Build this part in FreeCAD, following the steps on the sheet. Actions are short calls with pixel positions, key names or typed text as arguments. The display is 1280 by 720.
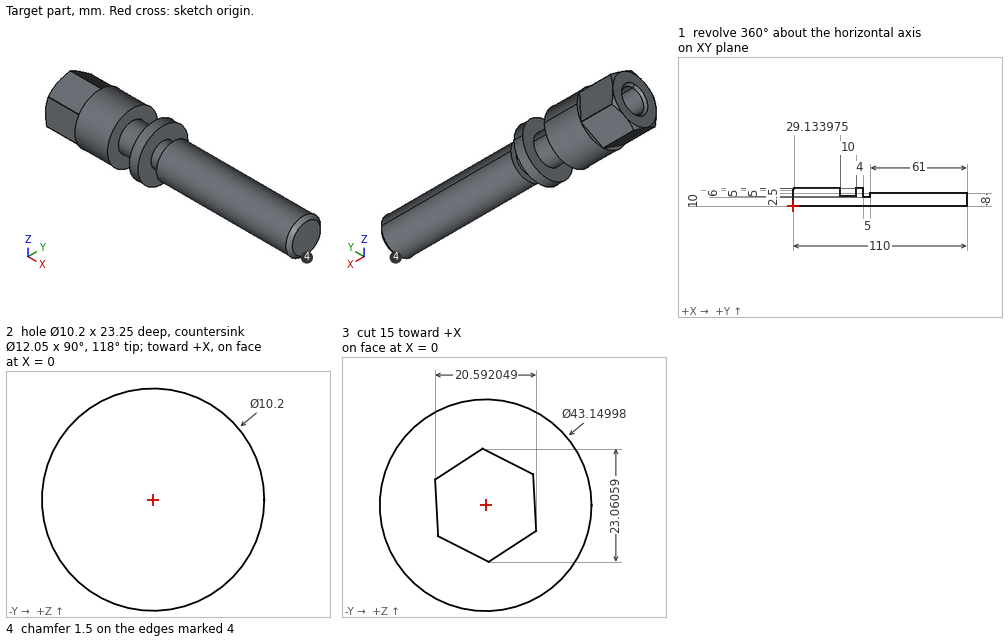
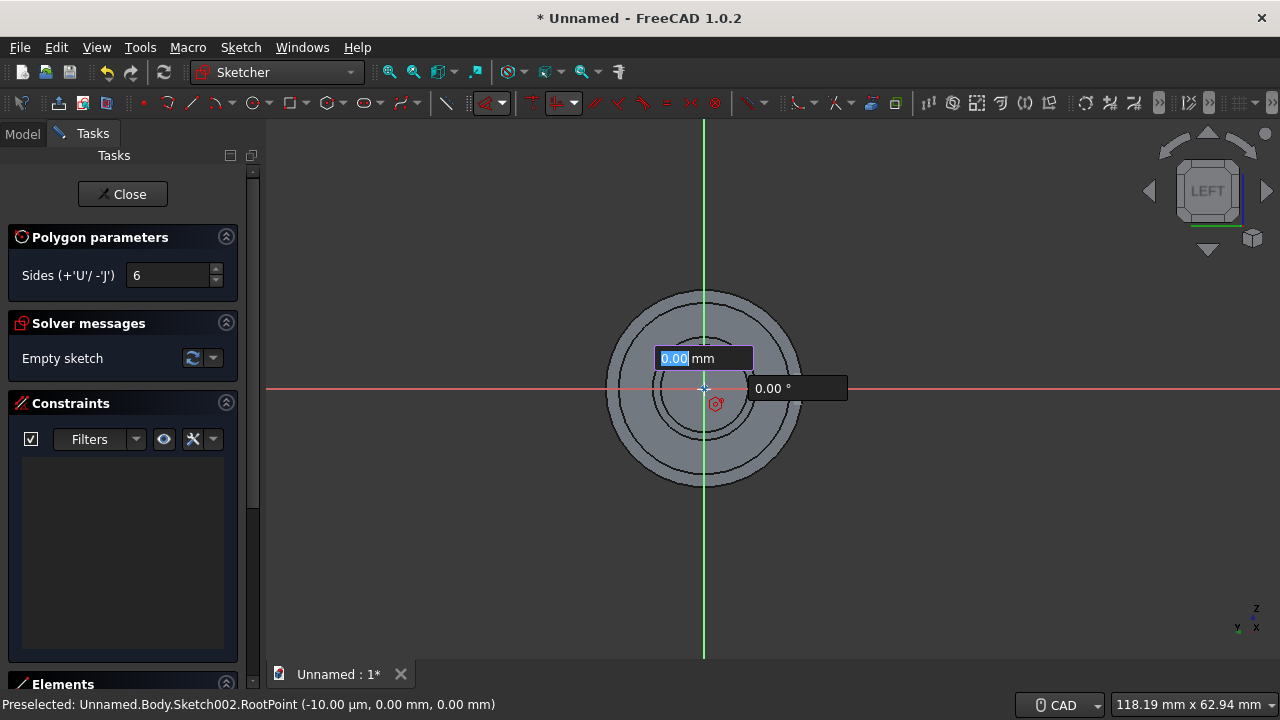
click(621, 443)
right_click(621, 443)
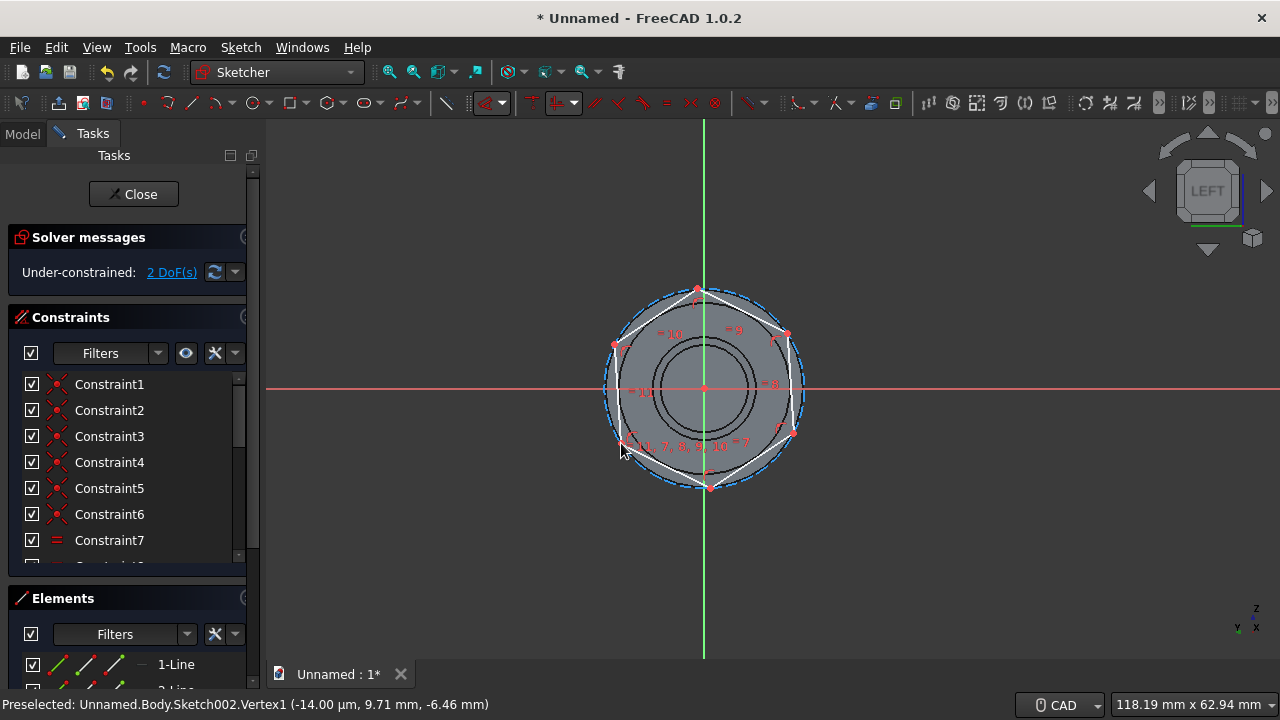
key(g)
key(c)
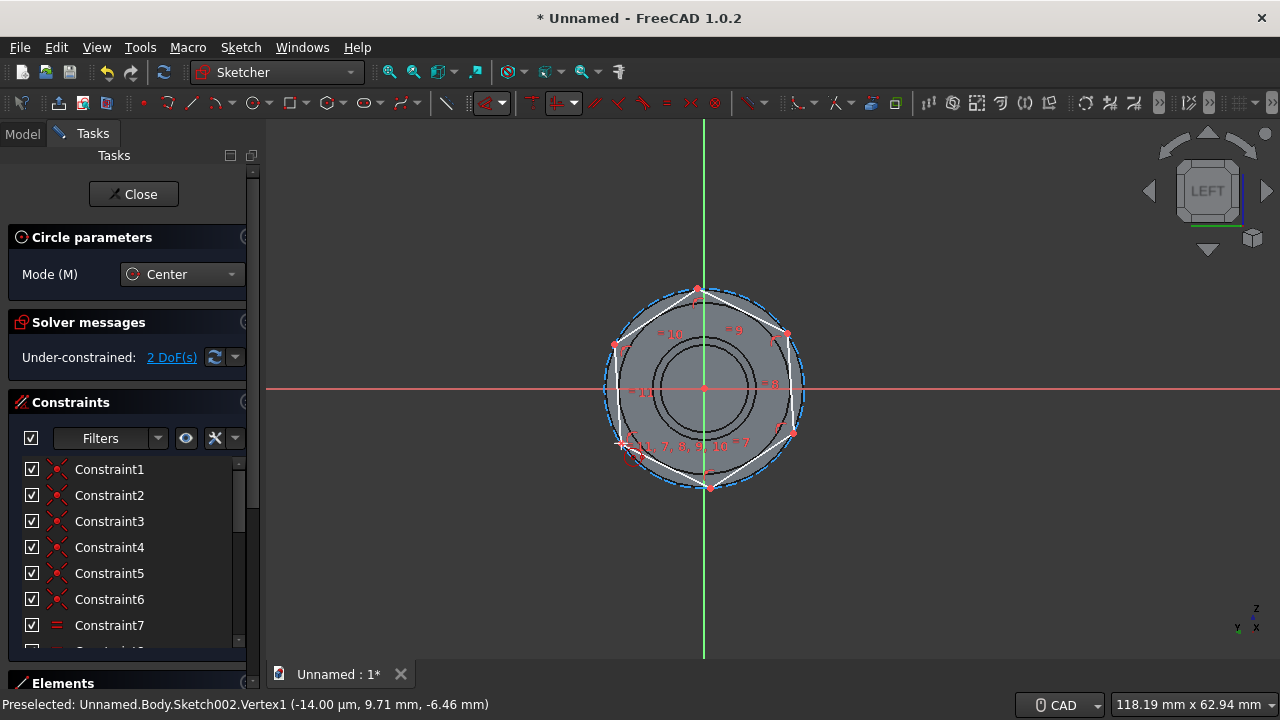
click(704, 389)
move(835, 258)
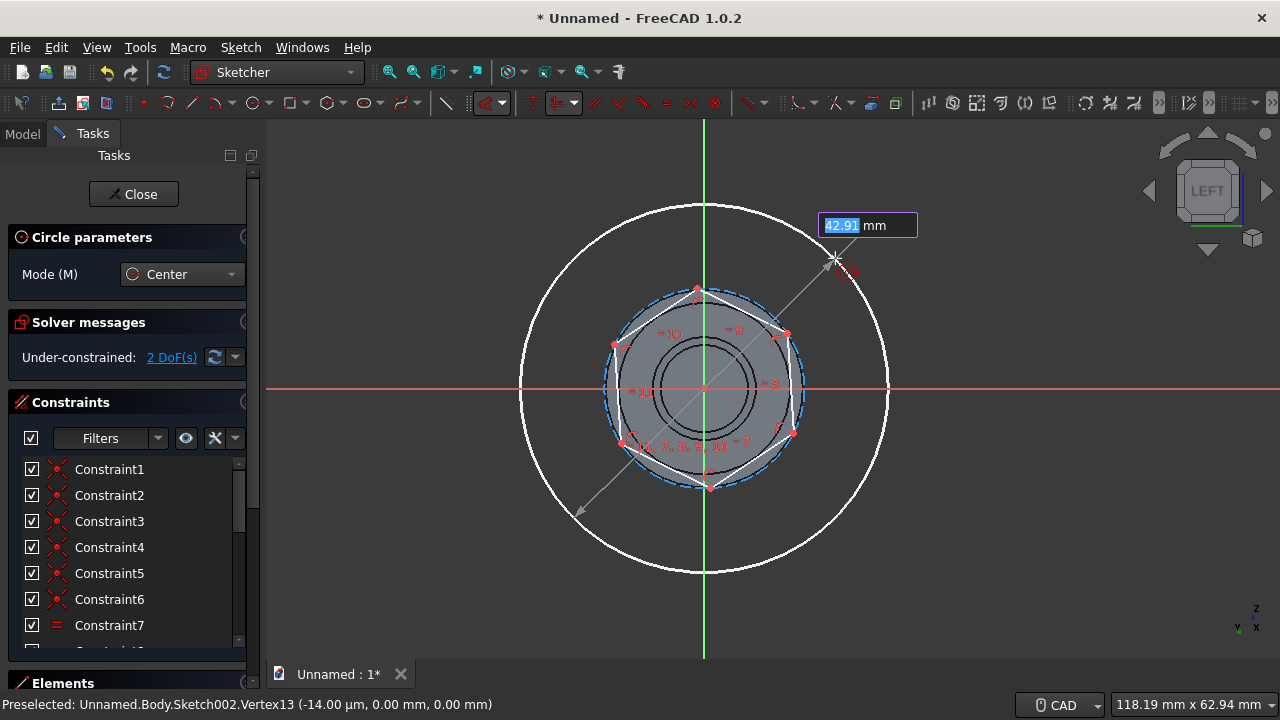
text(43.14998)
key(Return)
key(Escape)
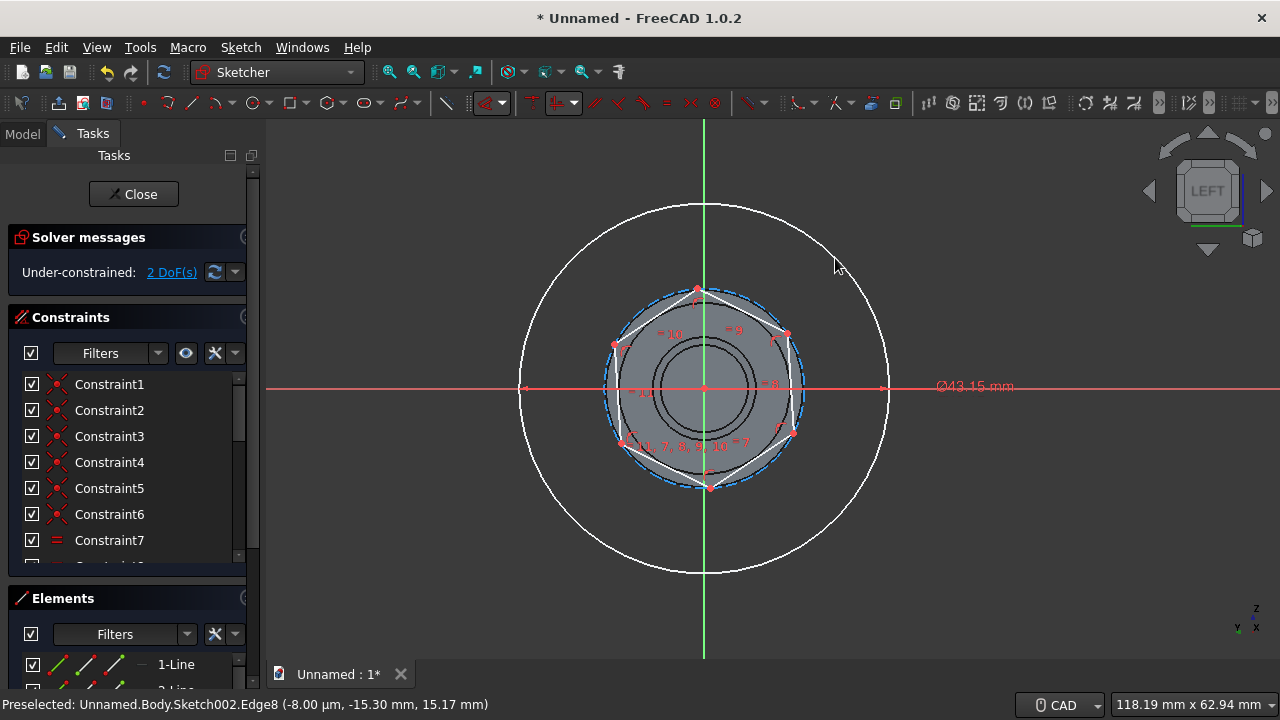
key(d)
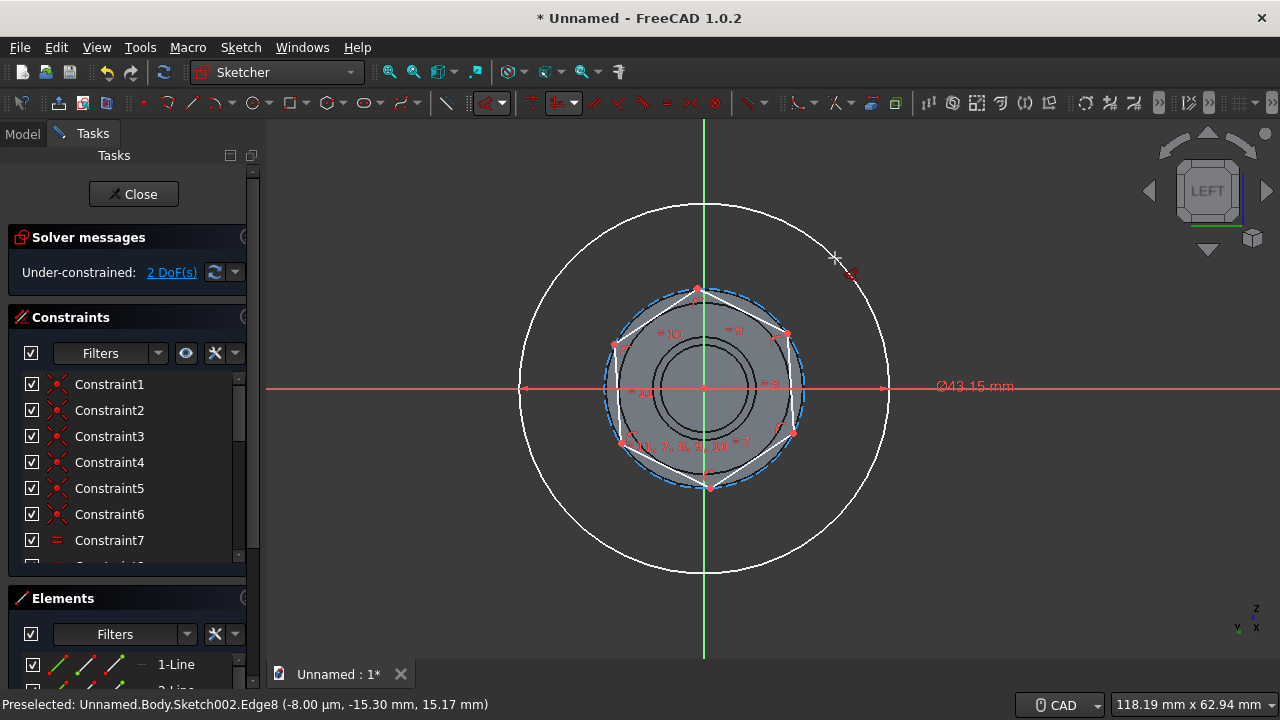
click(615, 344)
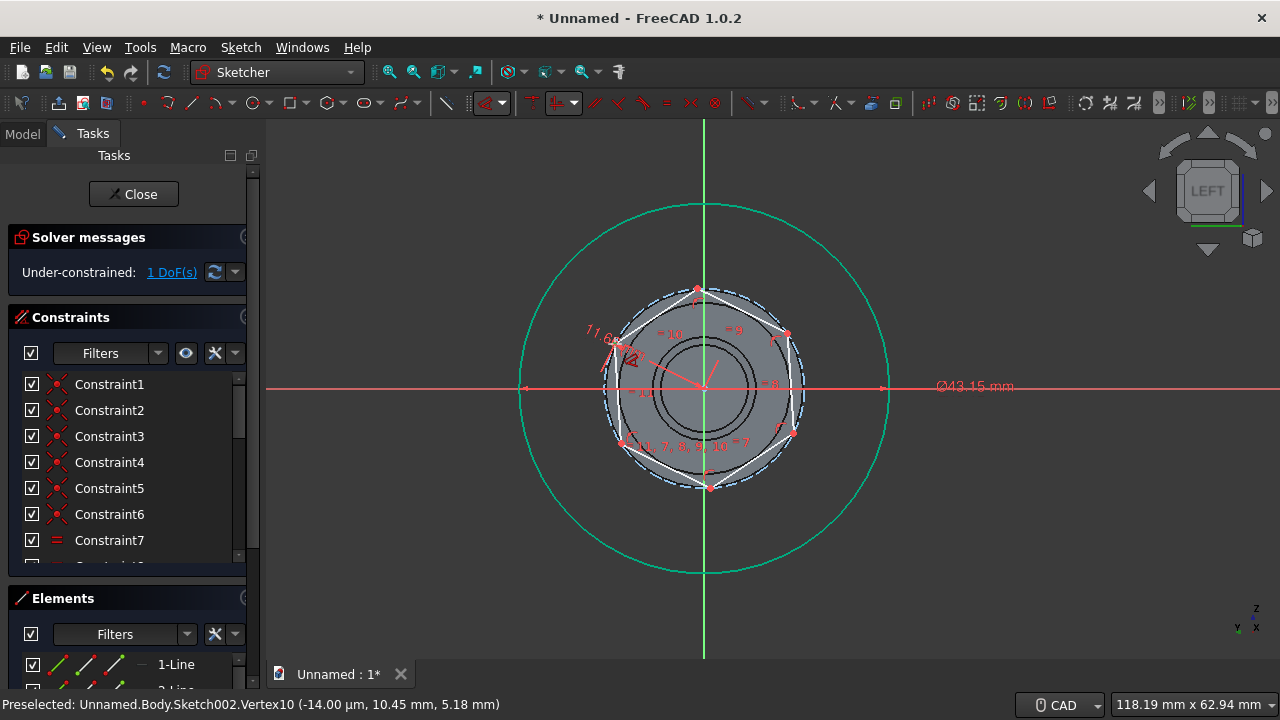
click(794, 433)
click(642, 286)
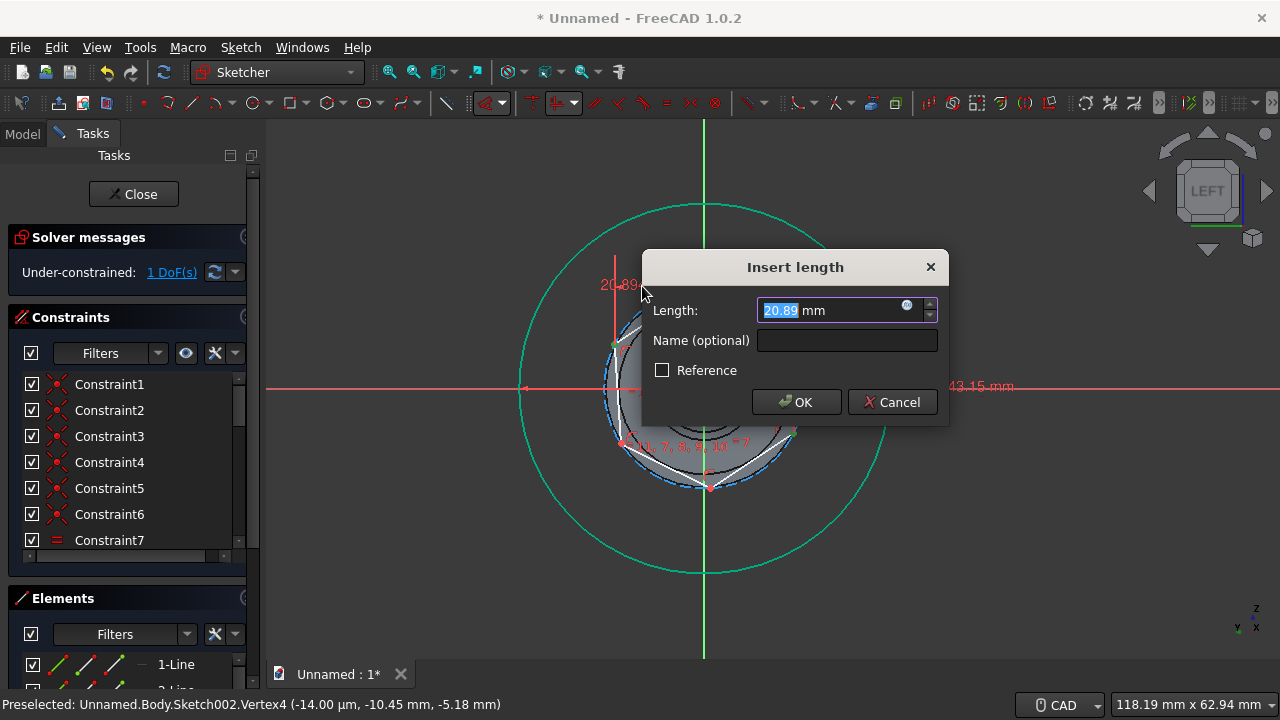
text(20.592049)
key(Return)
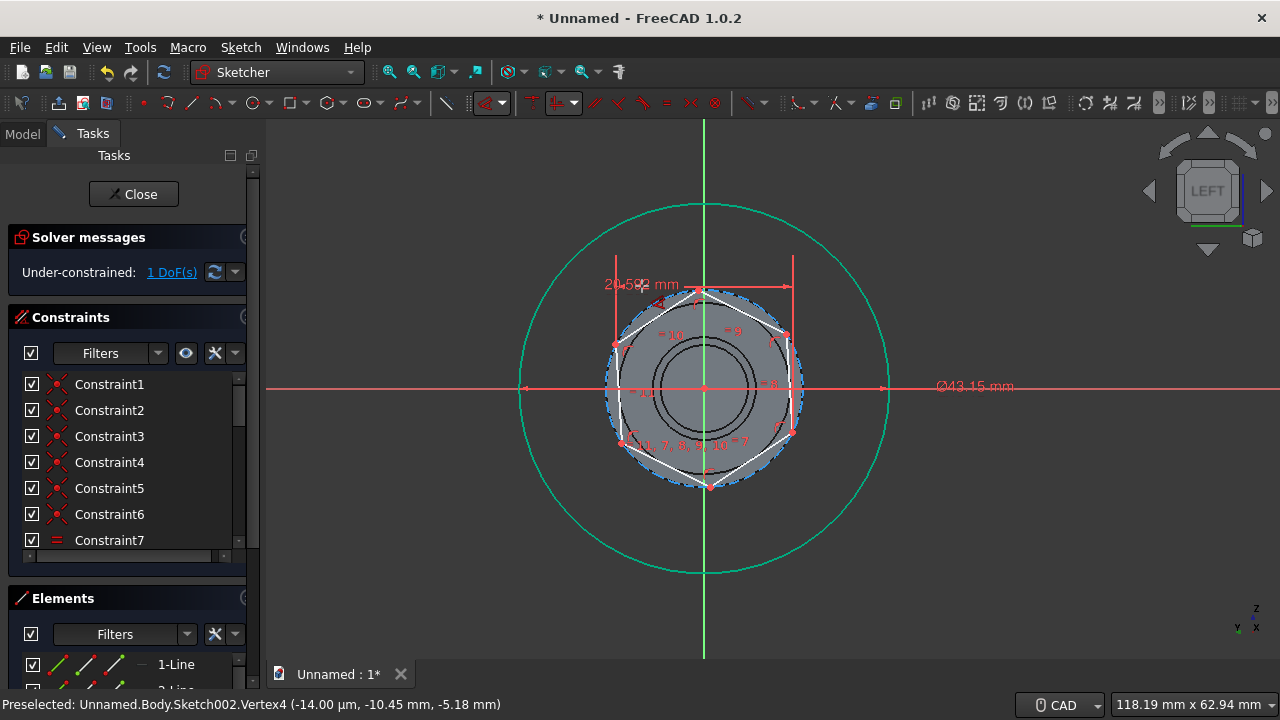
click(710, 487)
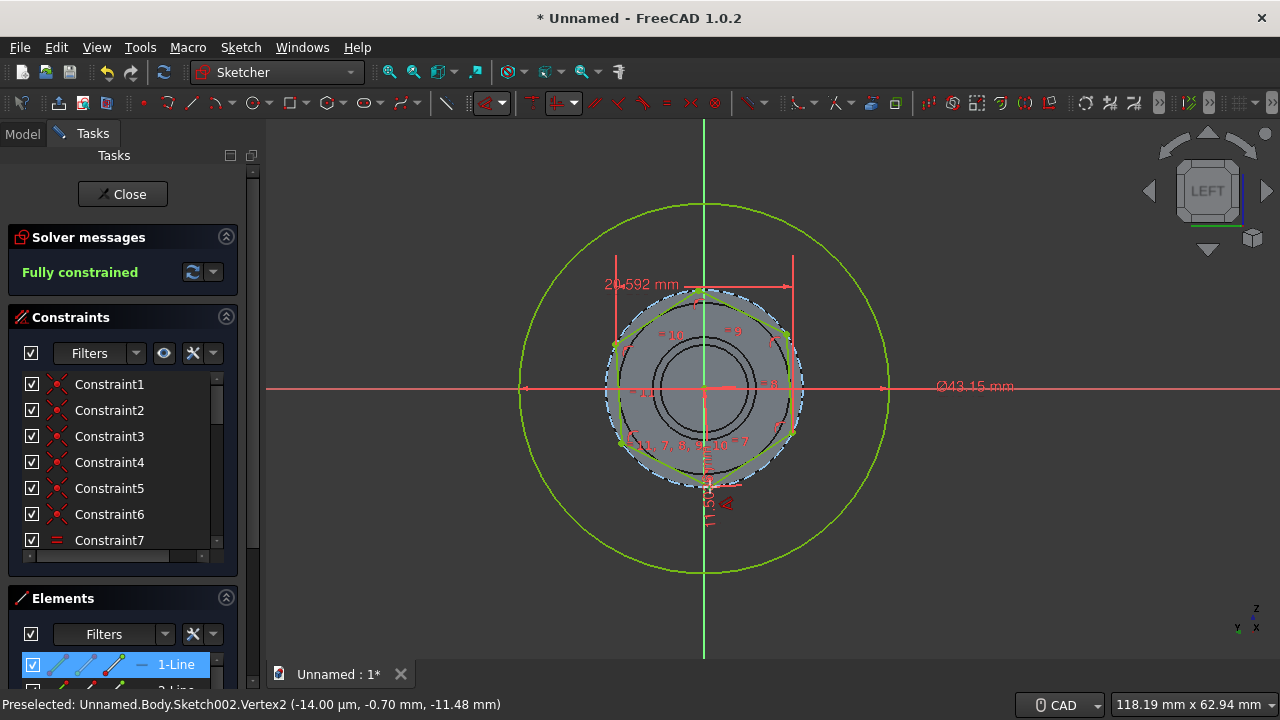
click(698, 290)
click(744, 343)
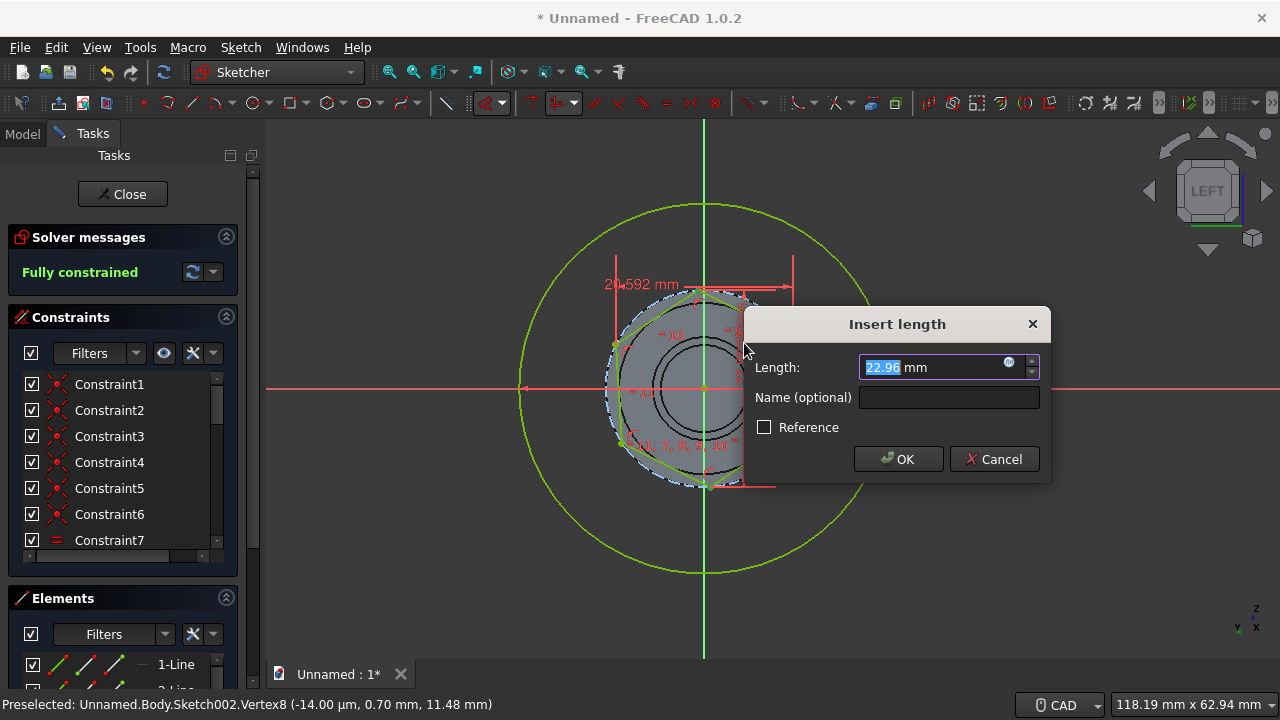
text(23.06059)
key(Return)
key(Escape)